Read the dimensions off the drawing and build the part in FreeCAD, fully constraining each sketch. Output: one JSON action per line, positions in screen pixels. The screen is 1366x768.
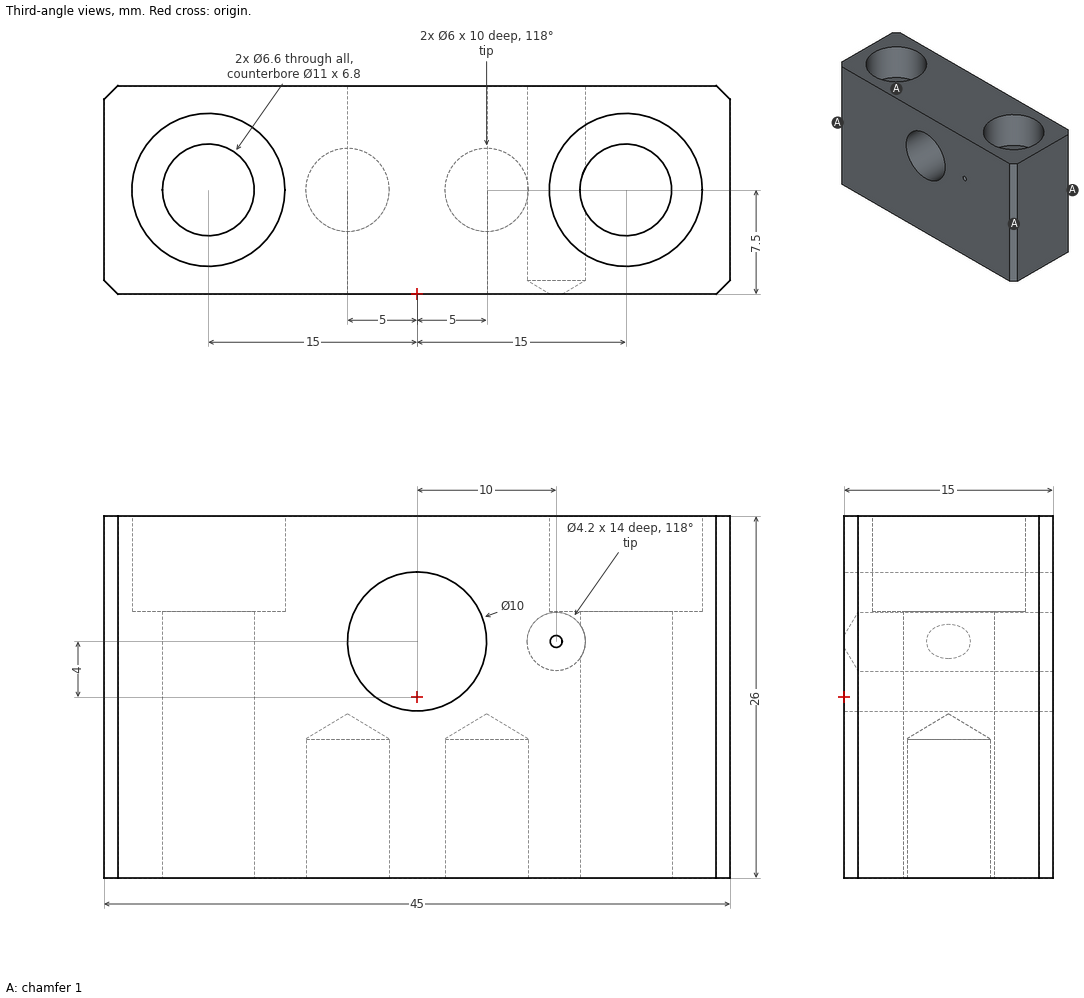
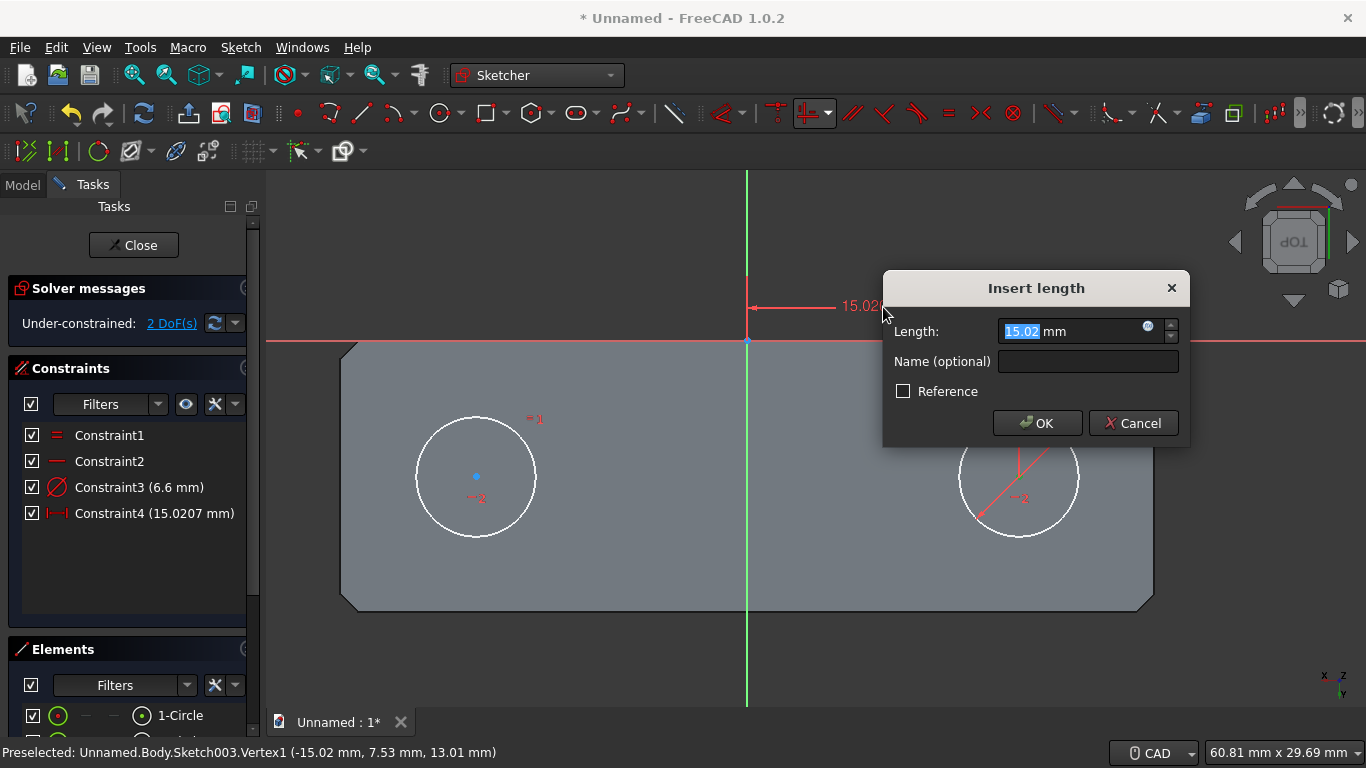
{"action": "type", "text": "15"}
{"action": "key", "text": "Return"}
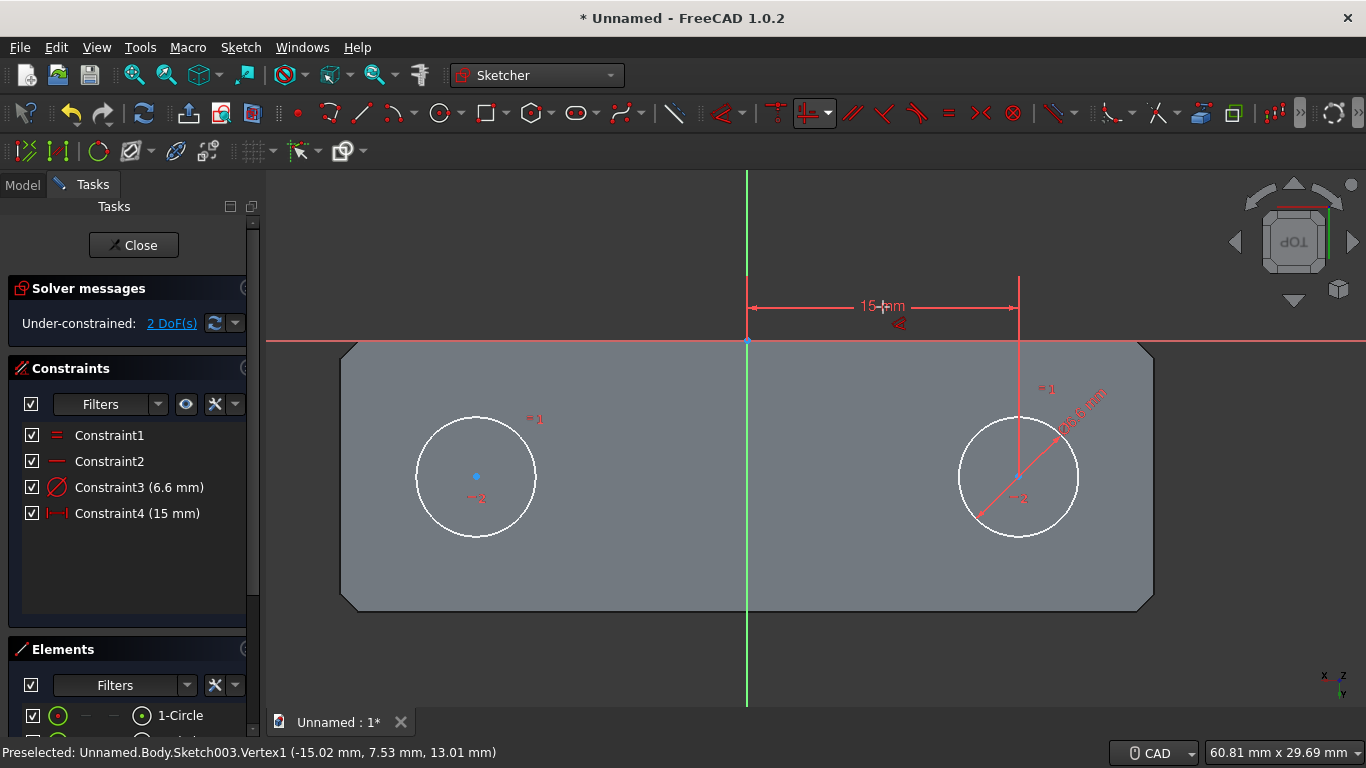
{"action": "left_click", "coordinate": [476, 477]}
{"action": "left_click", "coordinate": [612, 307]}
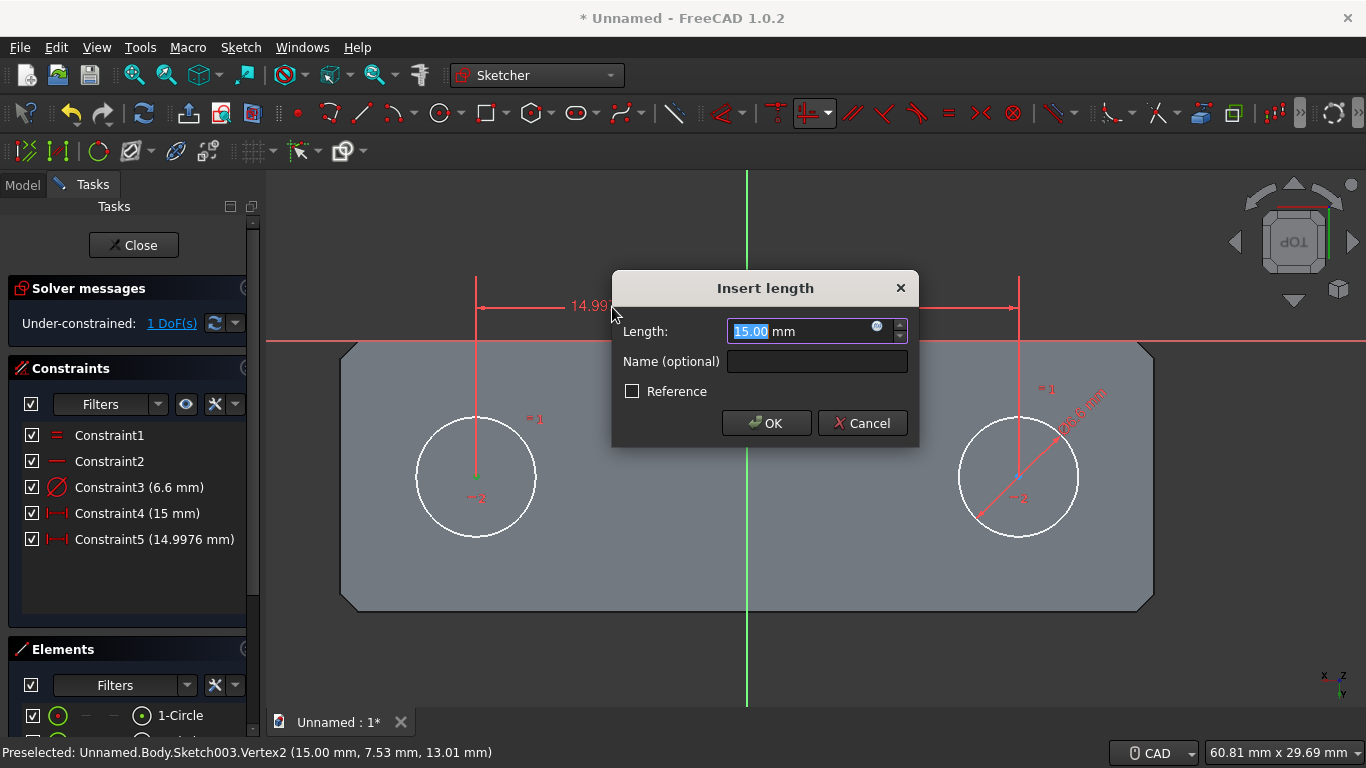
{"action": "type", "text": "15"}
{"action": "key", "text": "Return"}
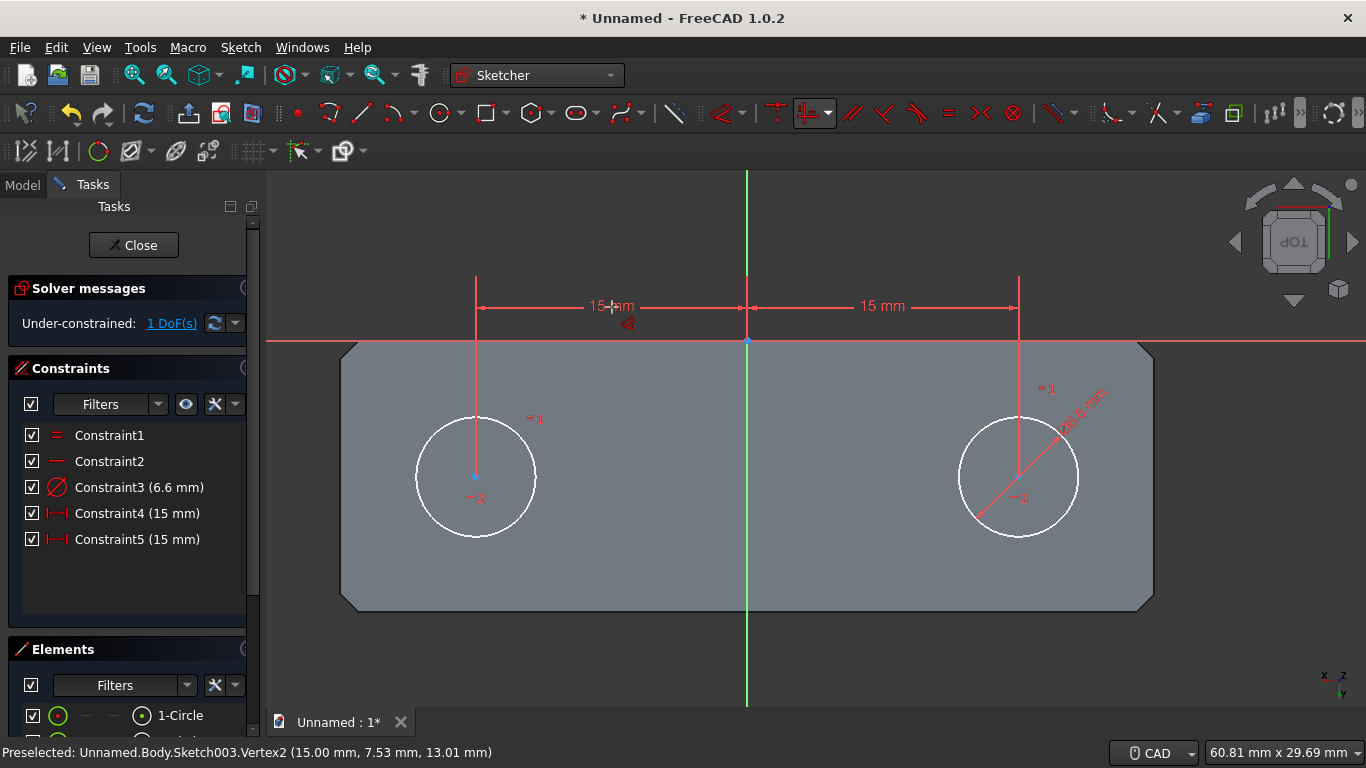
{"action": "left_click", "coordinate": [1019, 477]}
{"action": "left_click", "coordinate": [1053, 378]}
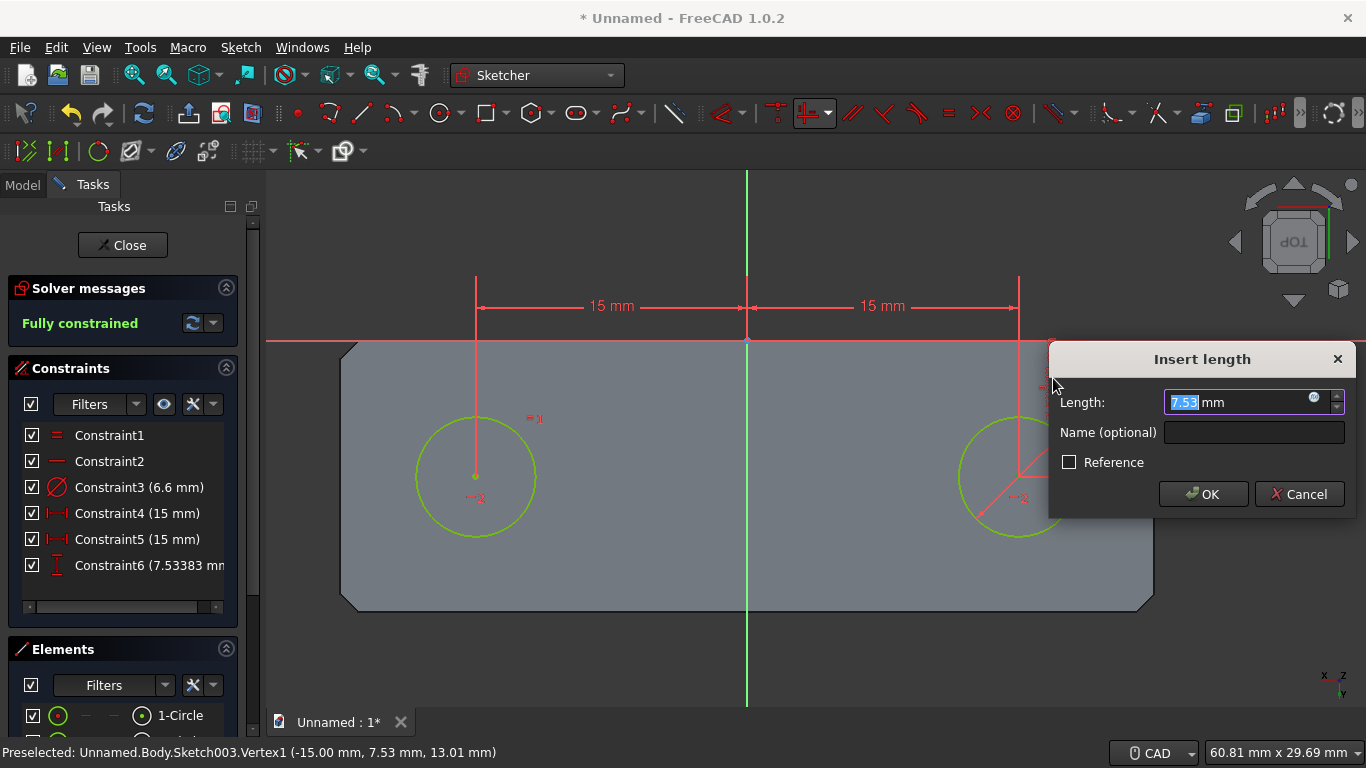
{"action": "type", "text": "7.5"}
{"action": "key", "text": "Return"}
{"action": "key", "text": "Escape"}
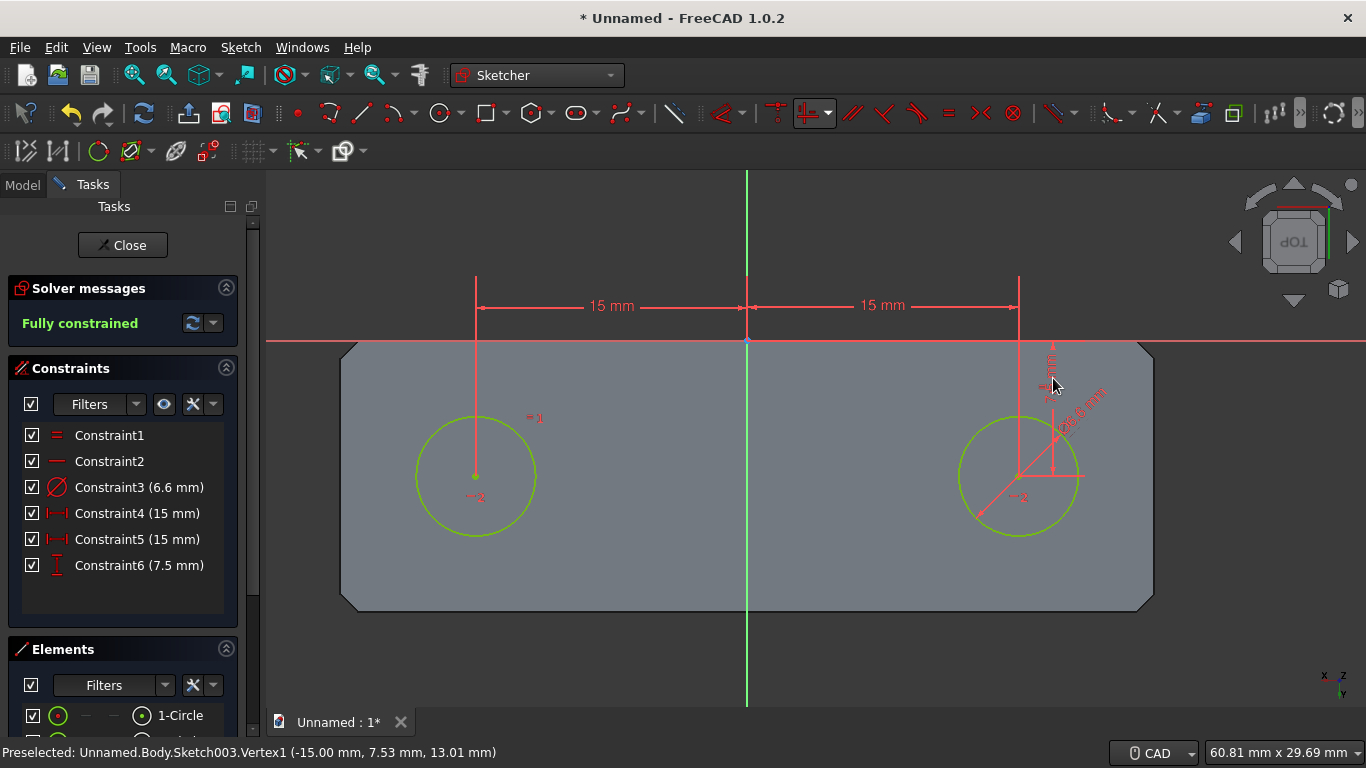
{"action": "left_click", "coordinate": [123, 245]}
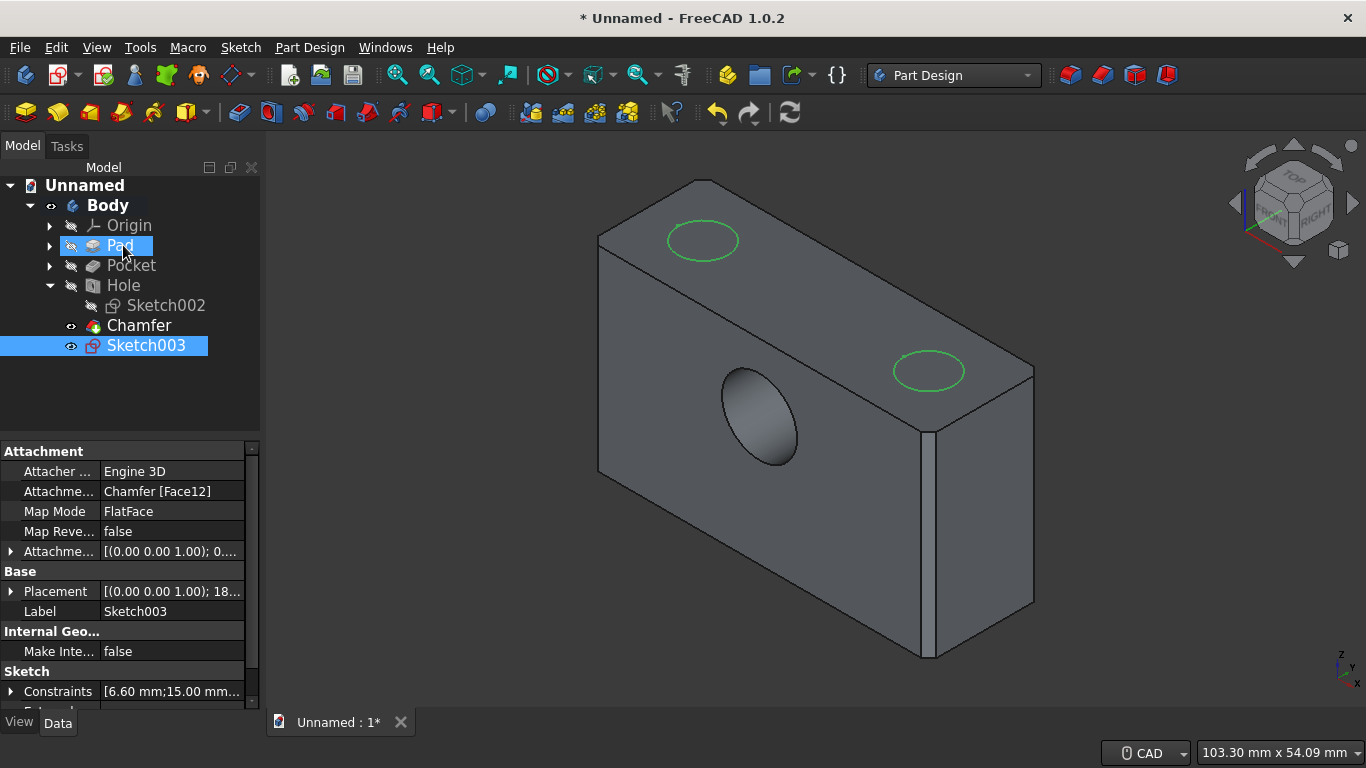
{"action": "left_click", "coordinate": [272, 112]}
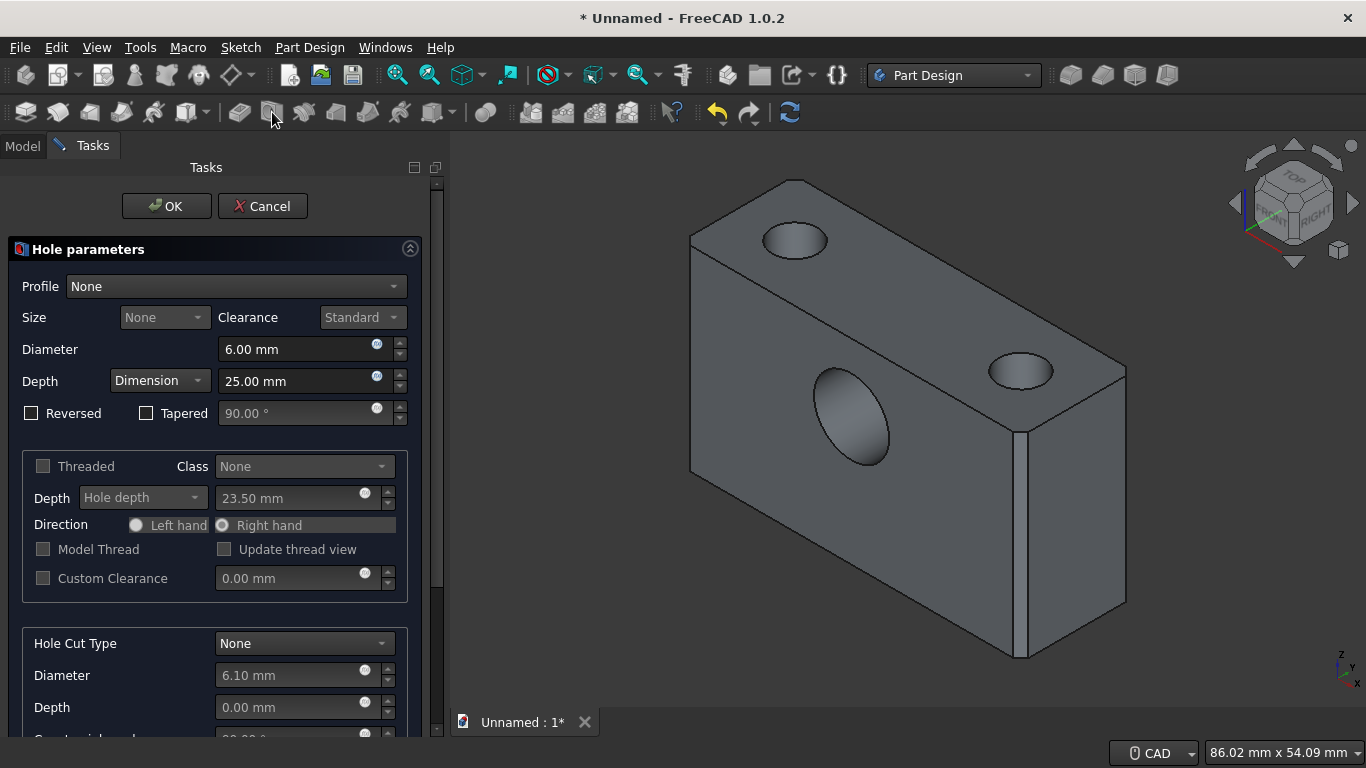
{"action": "triple_click", "coordinate": [305, 349]}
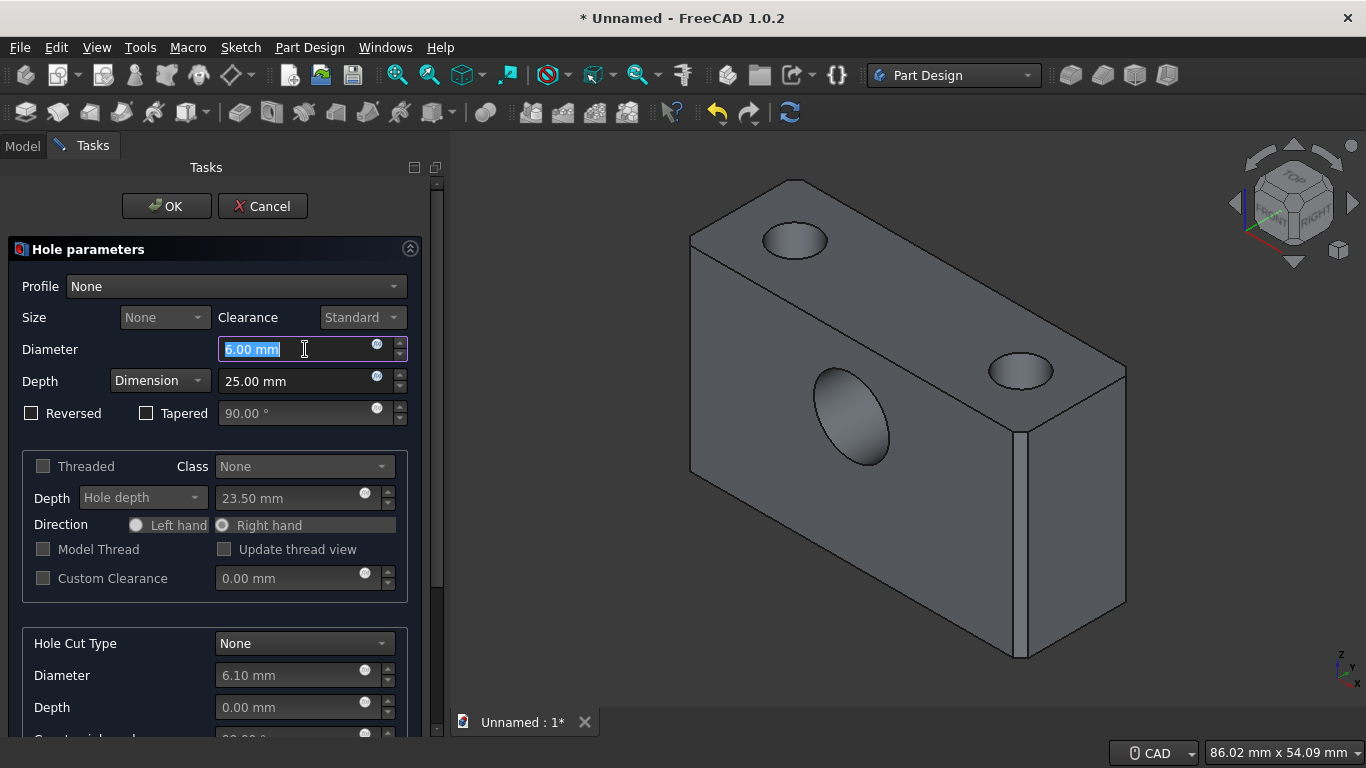
{"action": "type", "text": "6.6"}
{"action": "key", "text": "Tab"}